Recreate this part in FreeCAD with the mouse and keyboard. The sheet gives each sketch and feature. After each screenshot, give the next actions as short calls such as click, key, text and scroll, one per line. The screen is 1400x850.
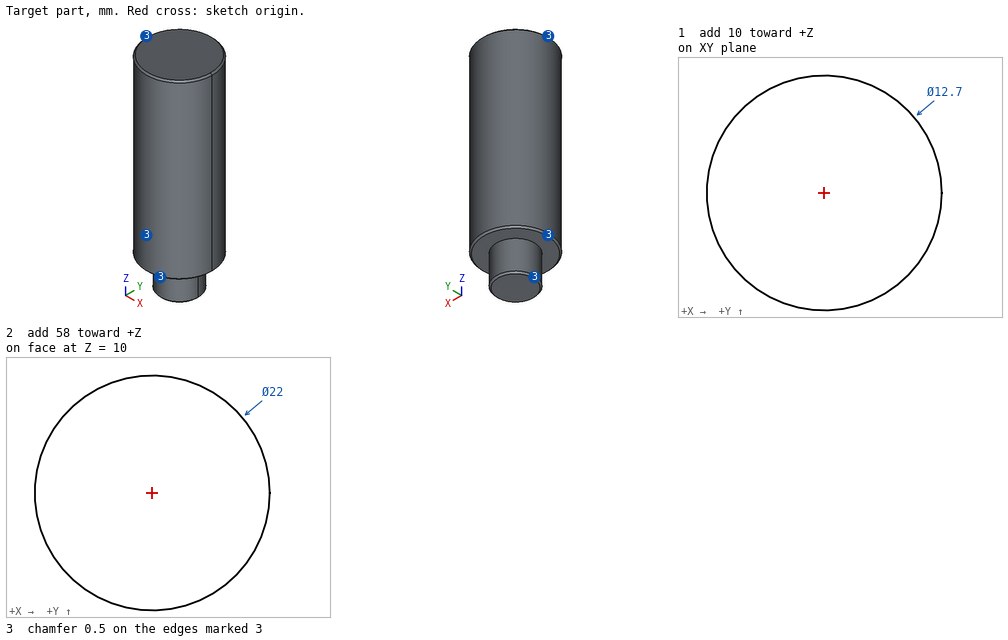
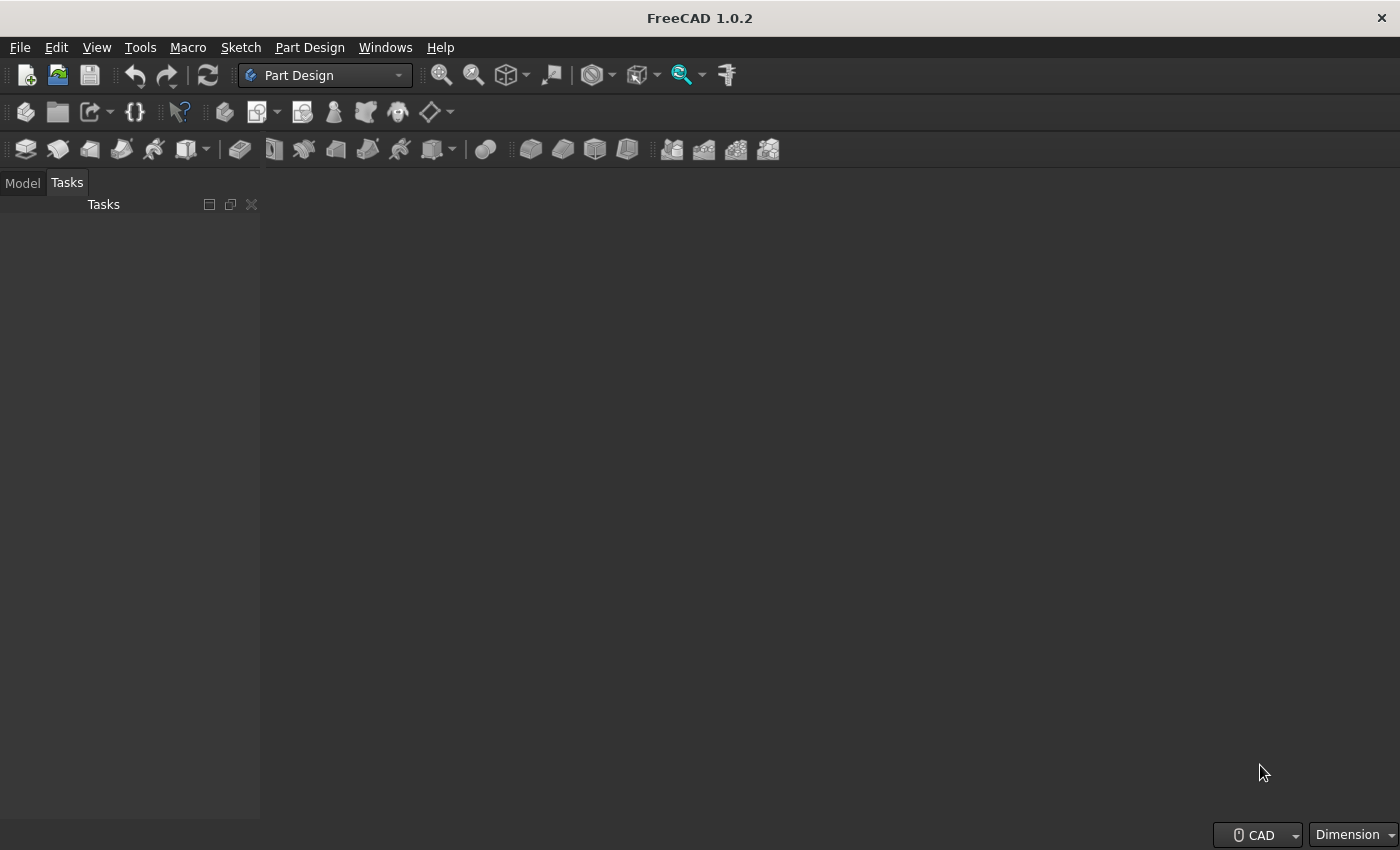
click(26, 76)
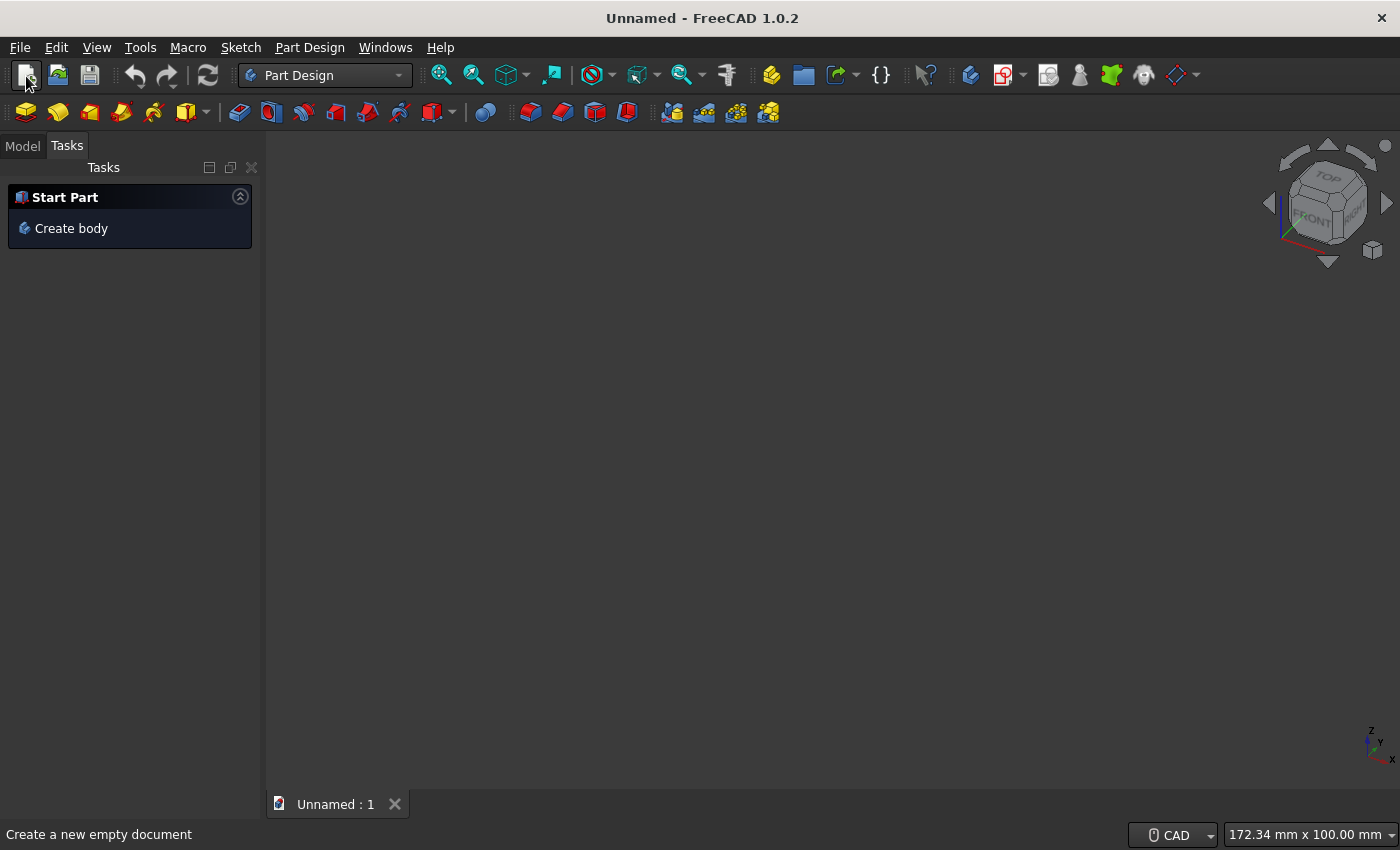
click(1004, 76)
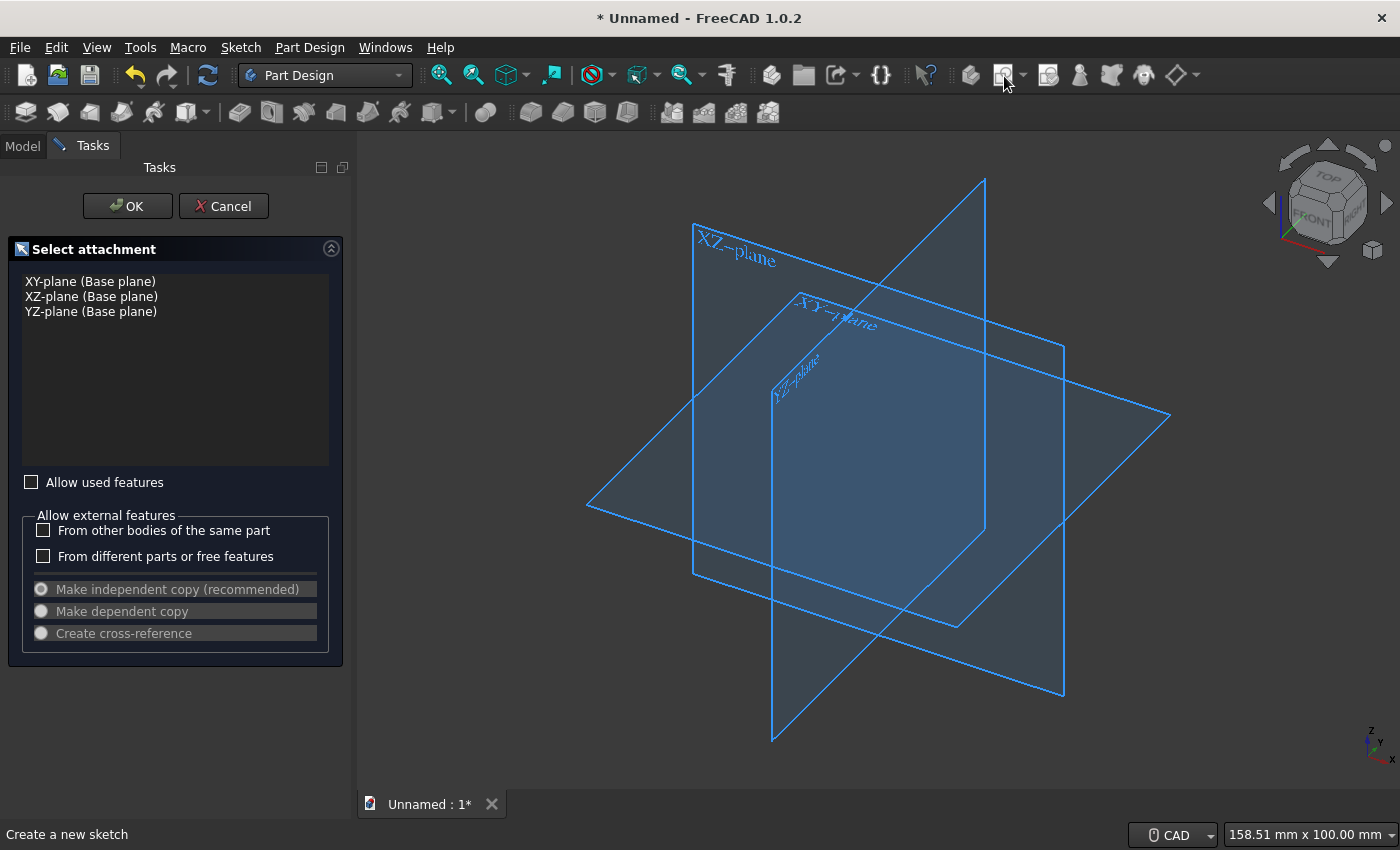
click(82, 282)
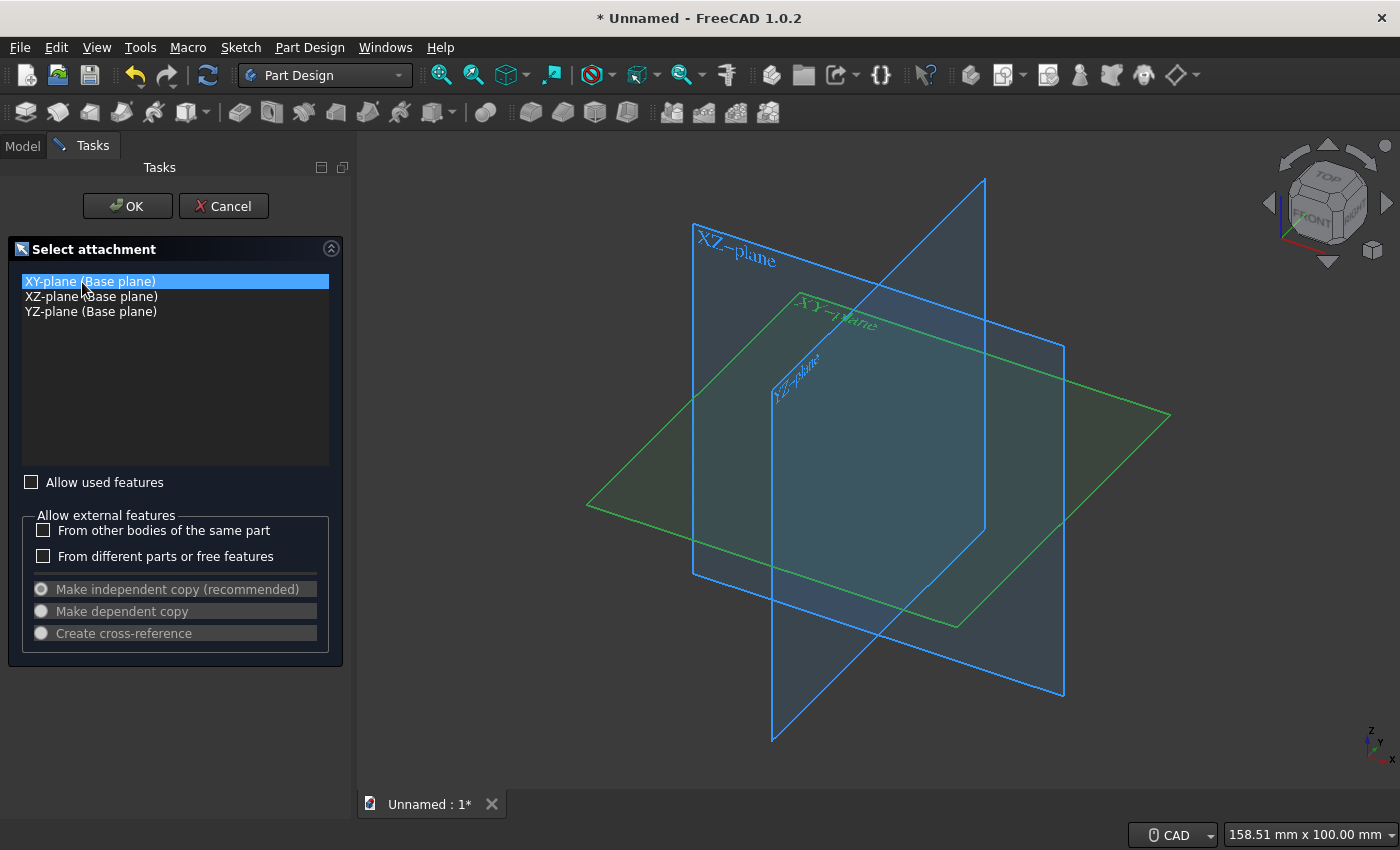
click(128, 206)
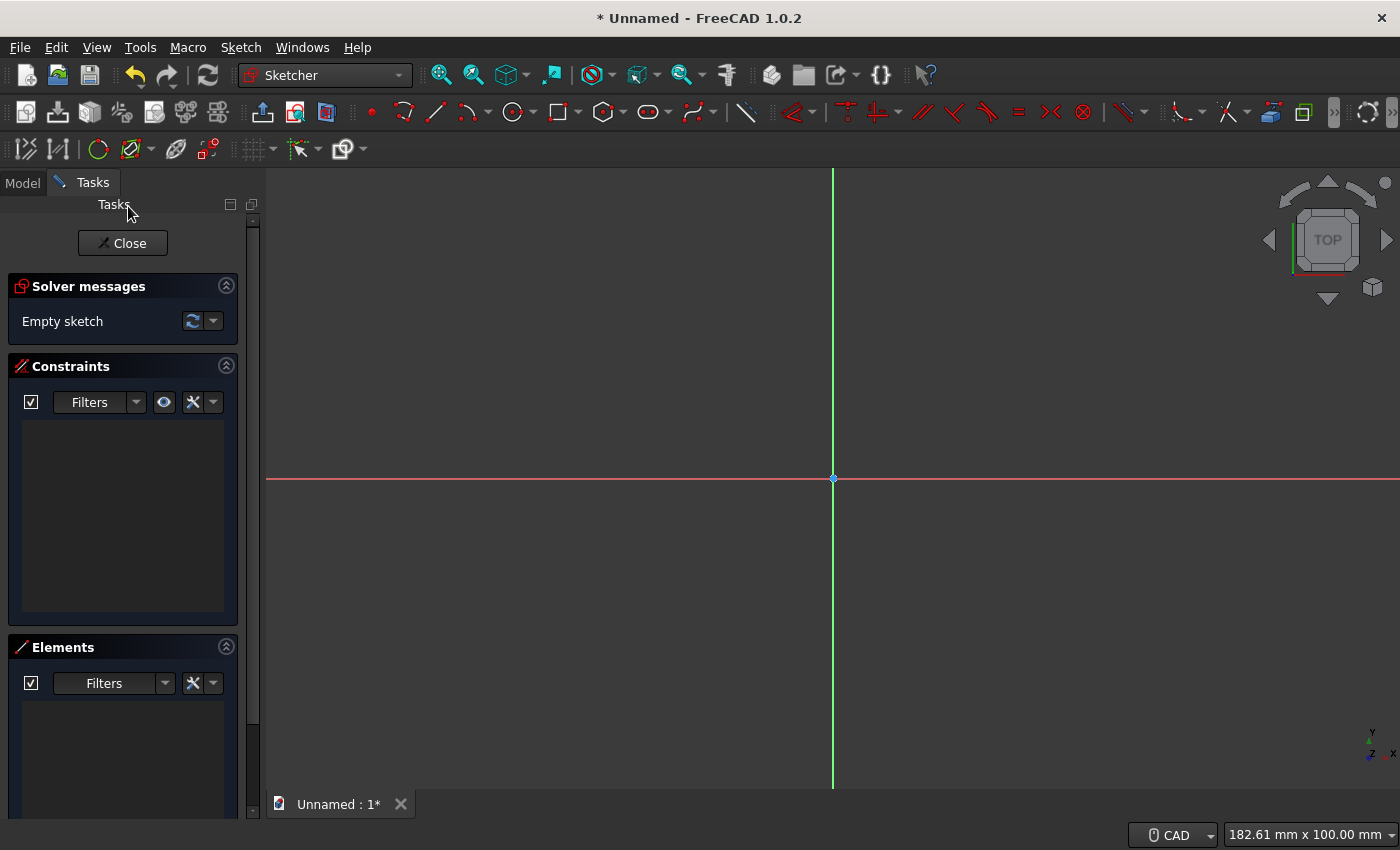
scroll(850, 478, up, 8)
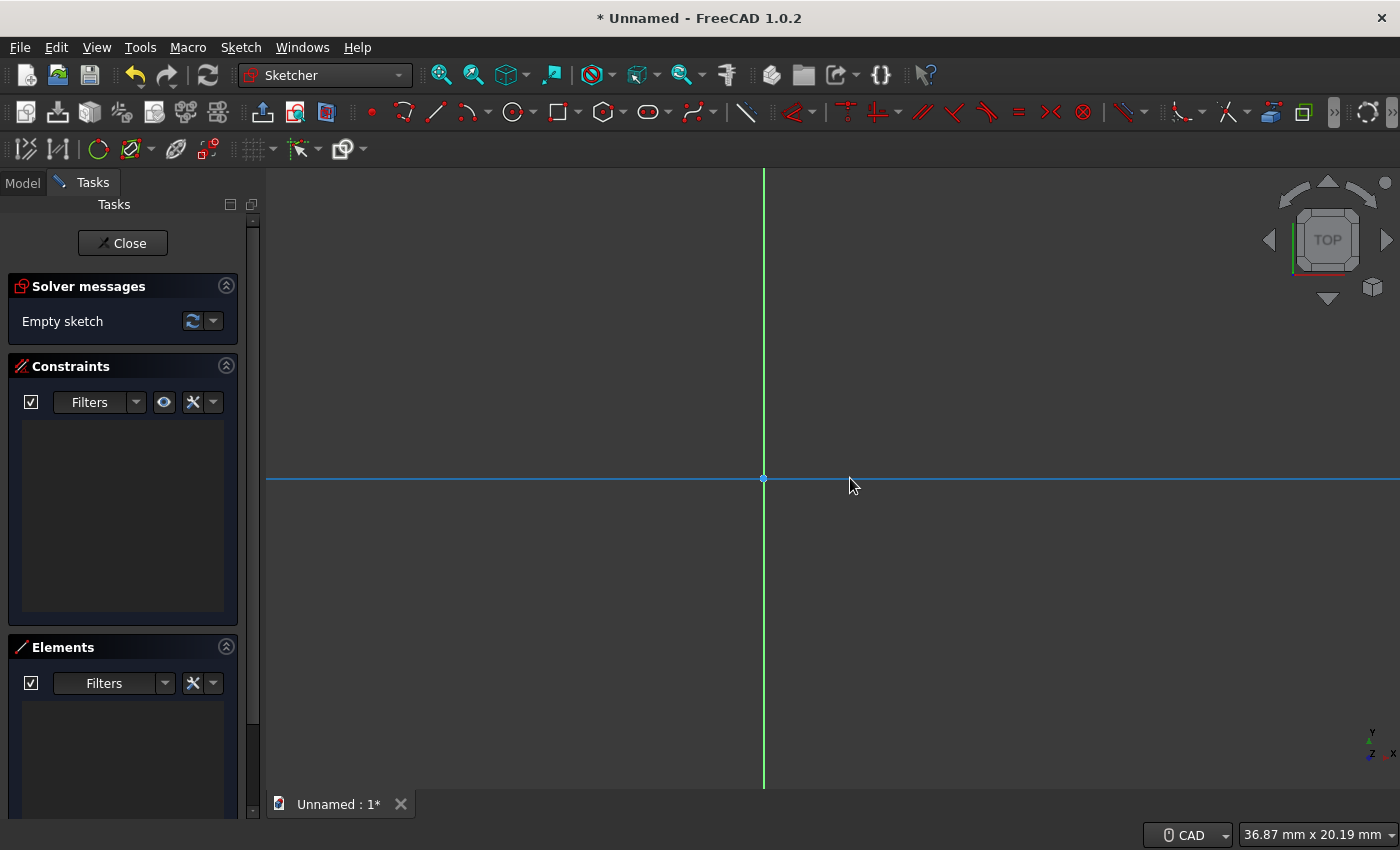
click(514, 112)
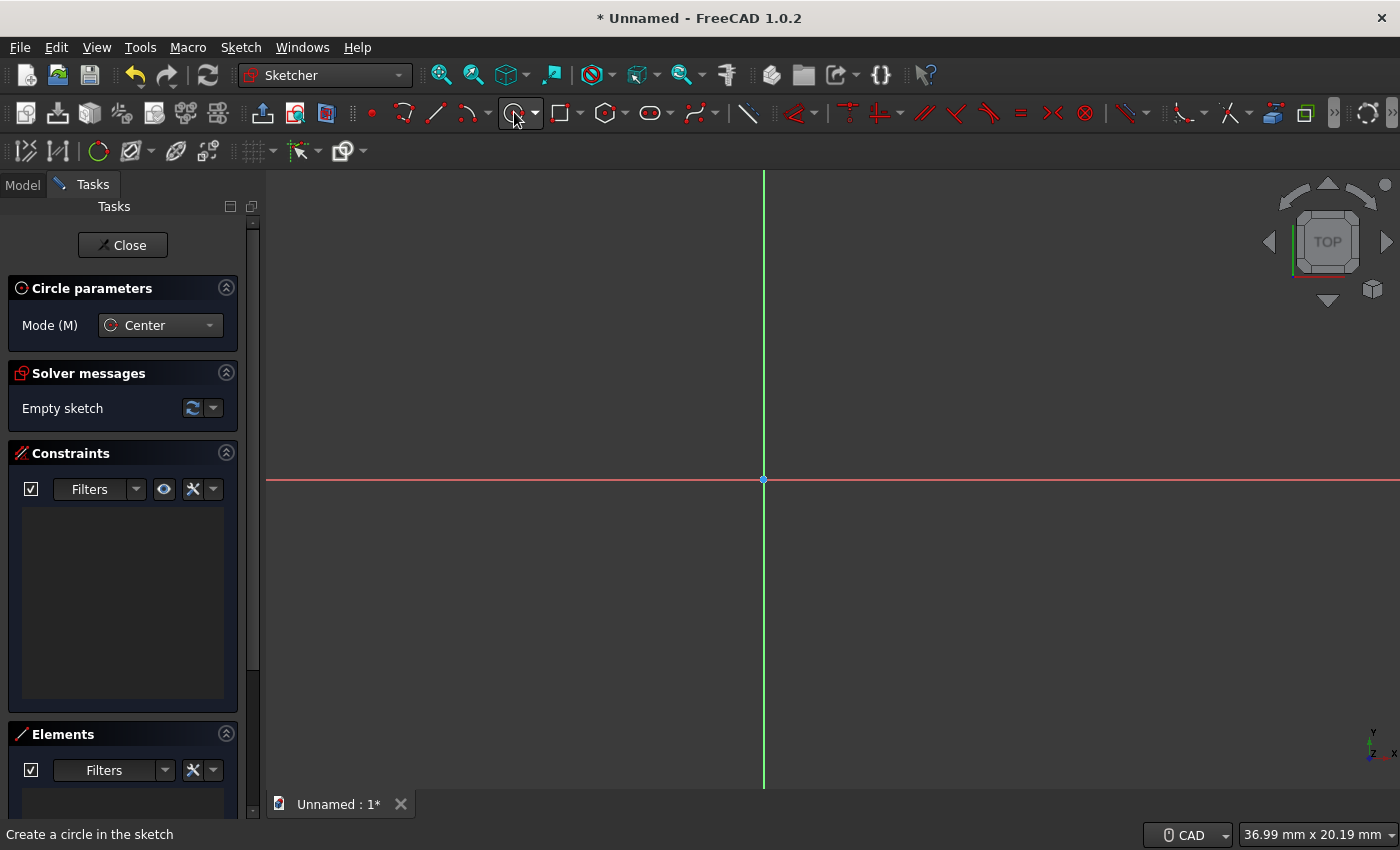
click(764, 480)
move(902, 342)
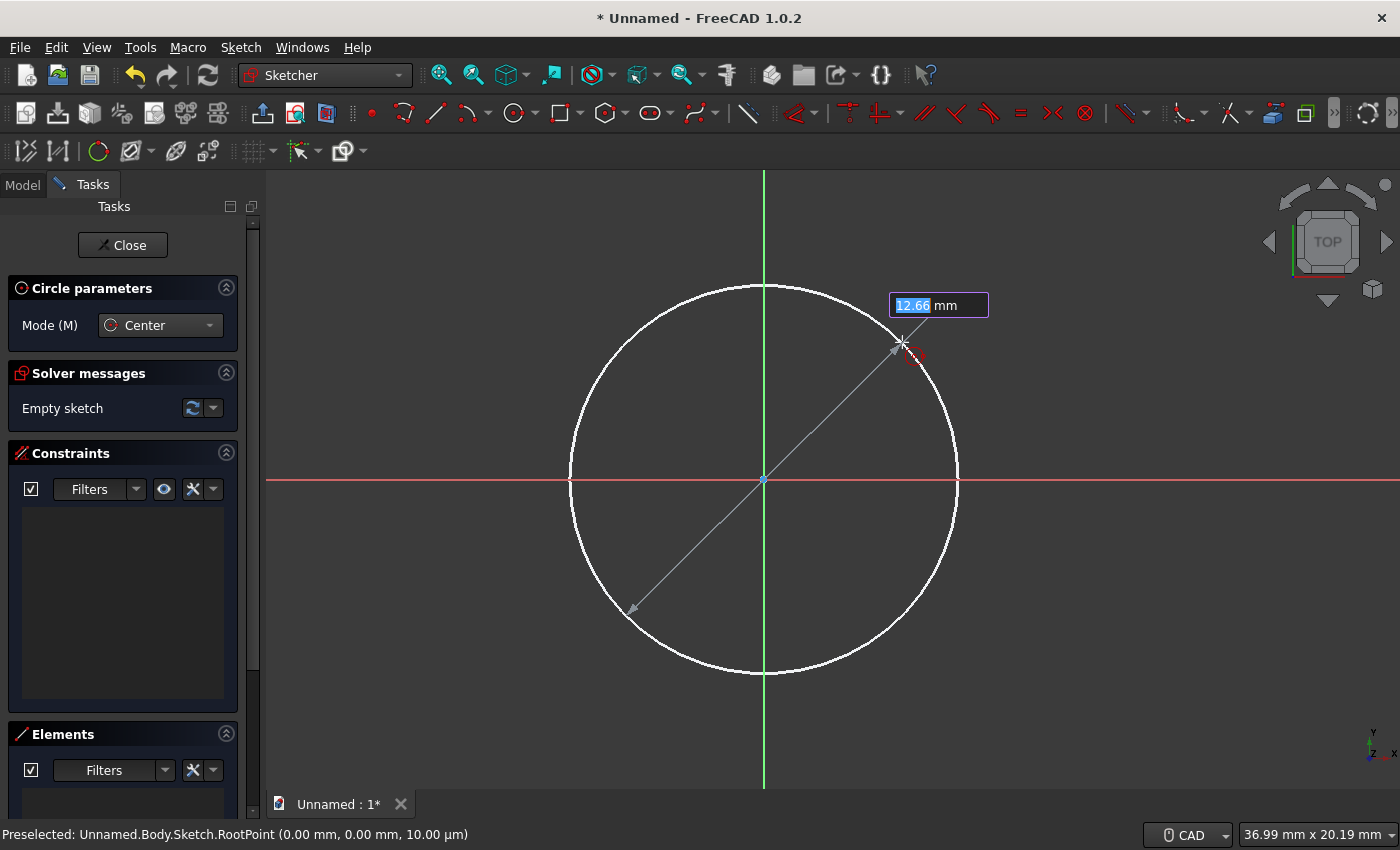
text(12.7)
key(Return)
key(Escape)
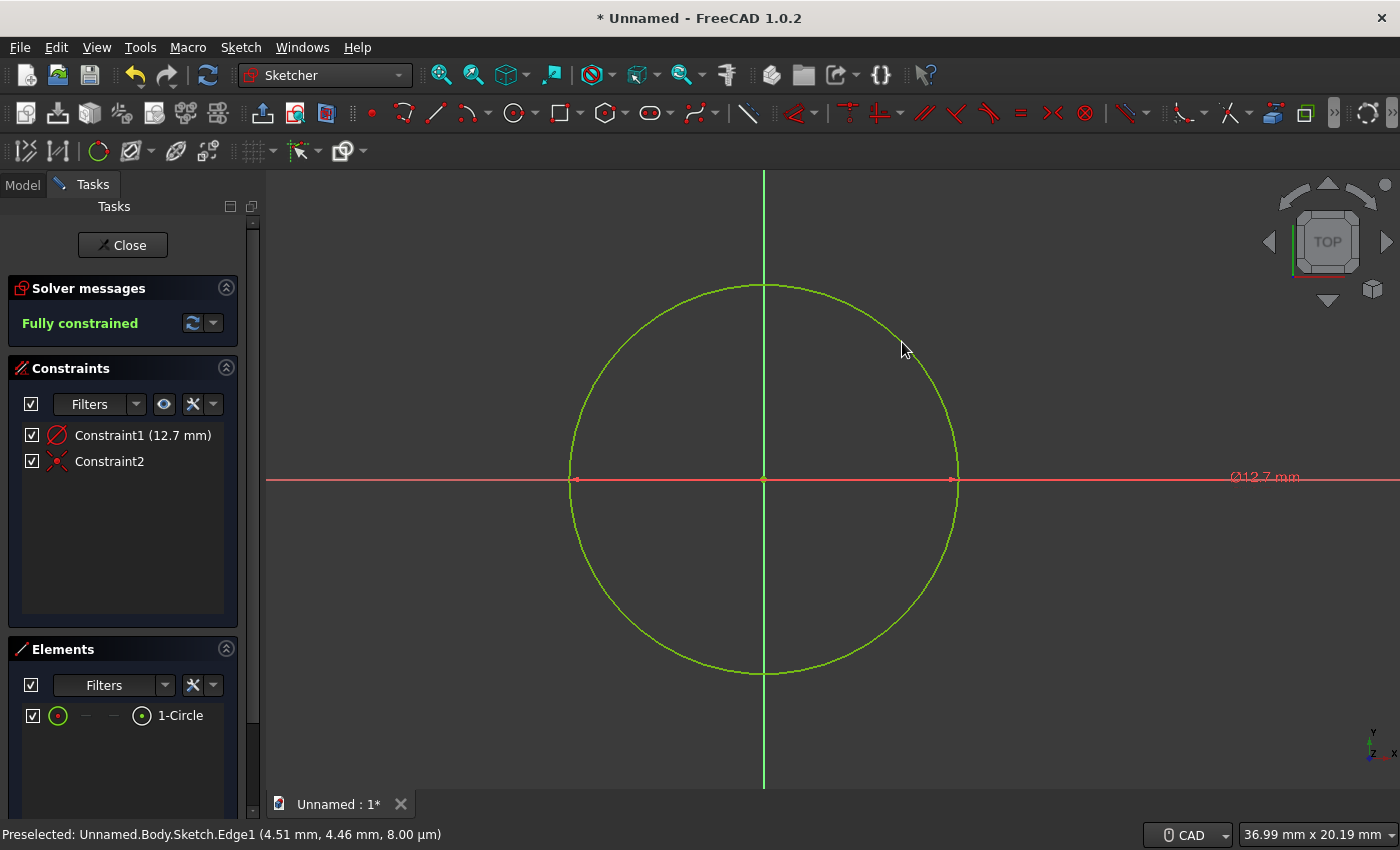
click(123, 245)